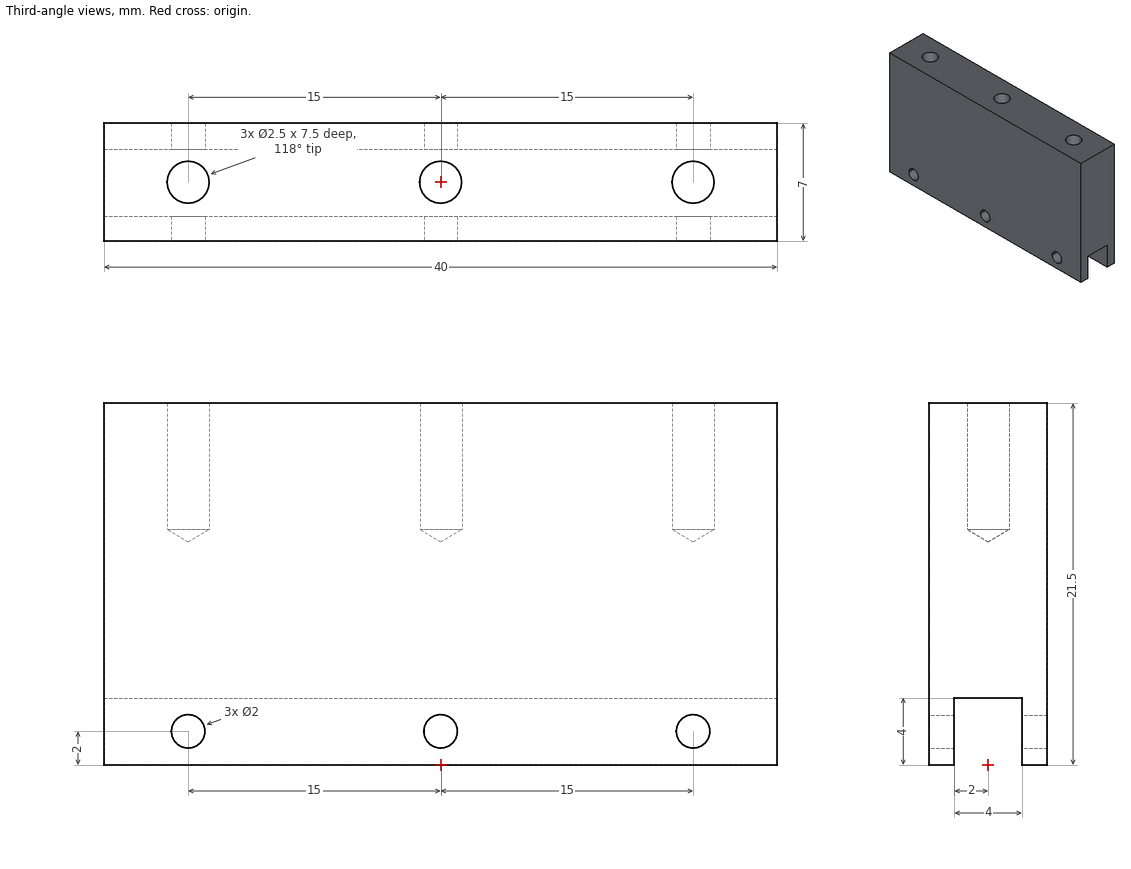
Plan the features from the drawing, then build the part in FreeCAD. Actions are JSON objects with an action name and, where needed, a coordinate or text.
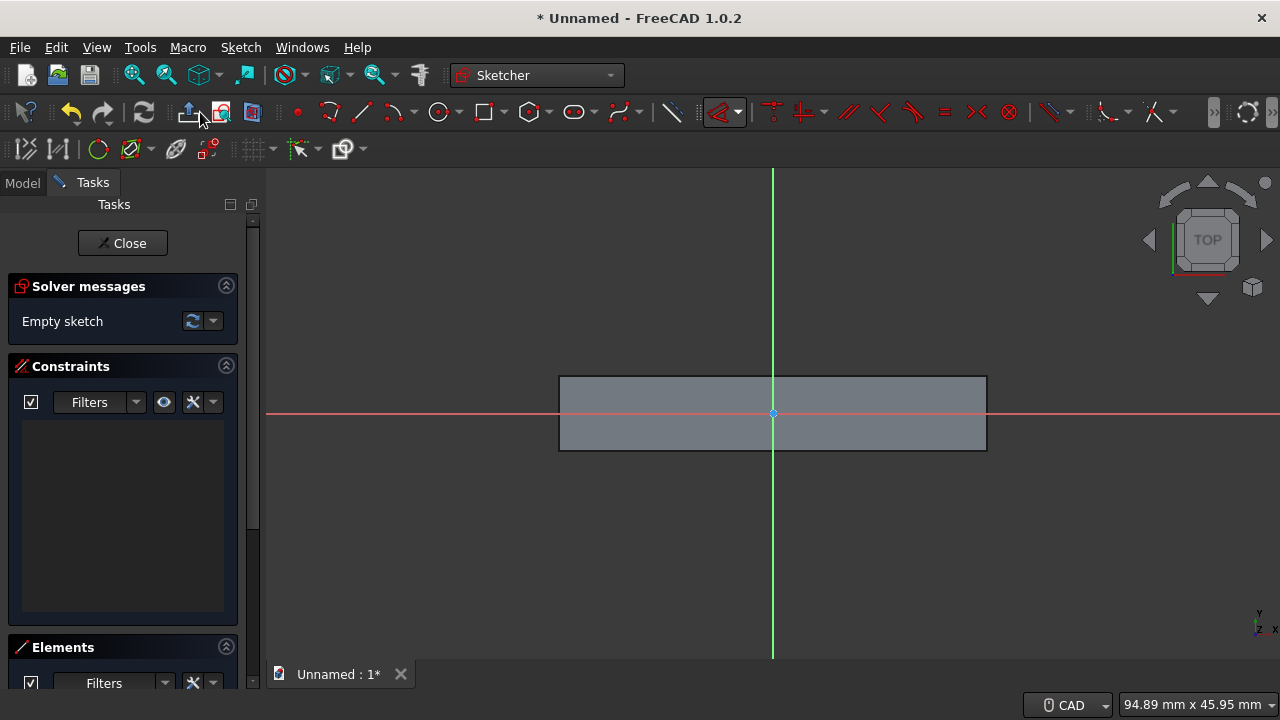
{"action": "scroll", "coordinate": [856, 414], "scroll_direction": "up", "scroll_amount": 3}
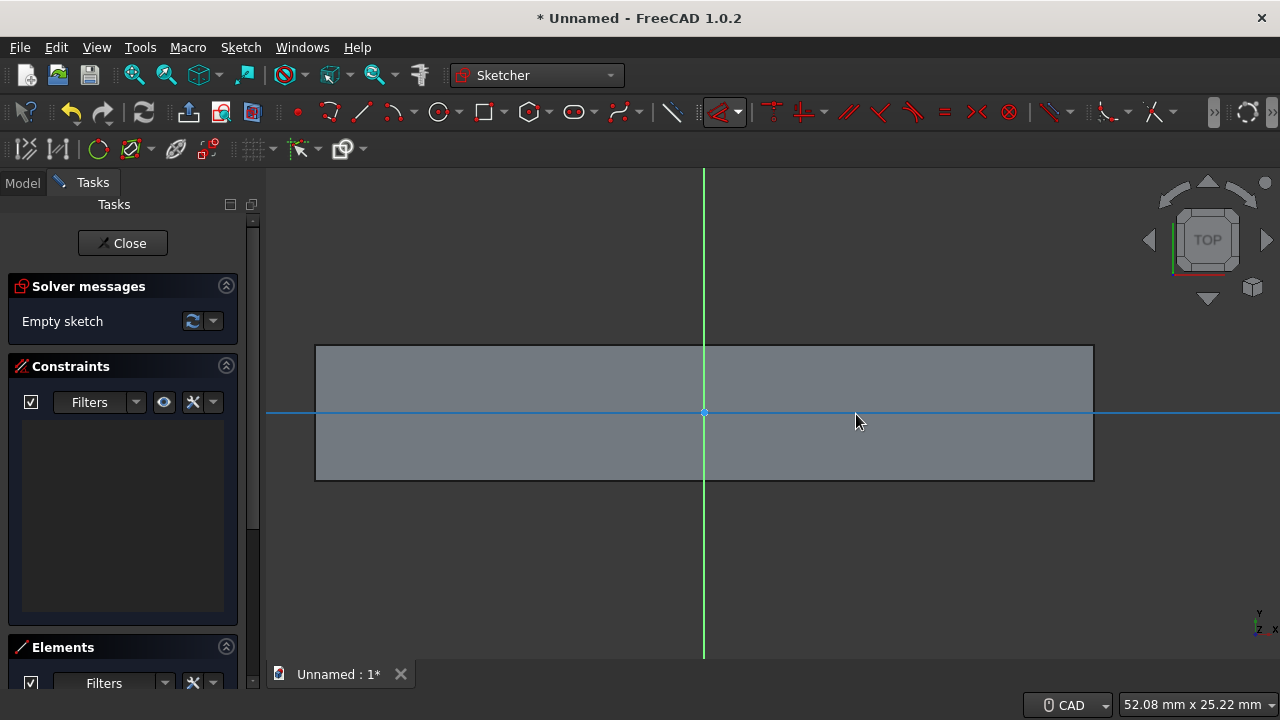
{"action": "left_click", "coordinate": [440, 112]}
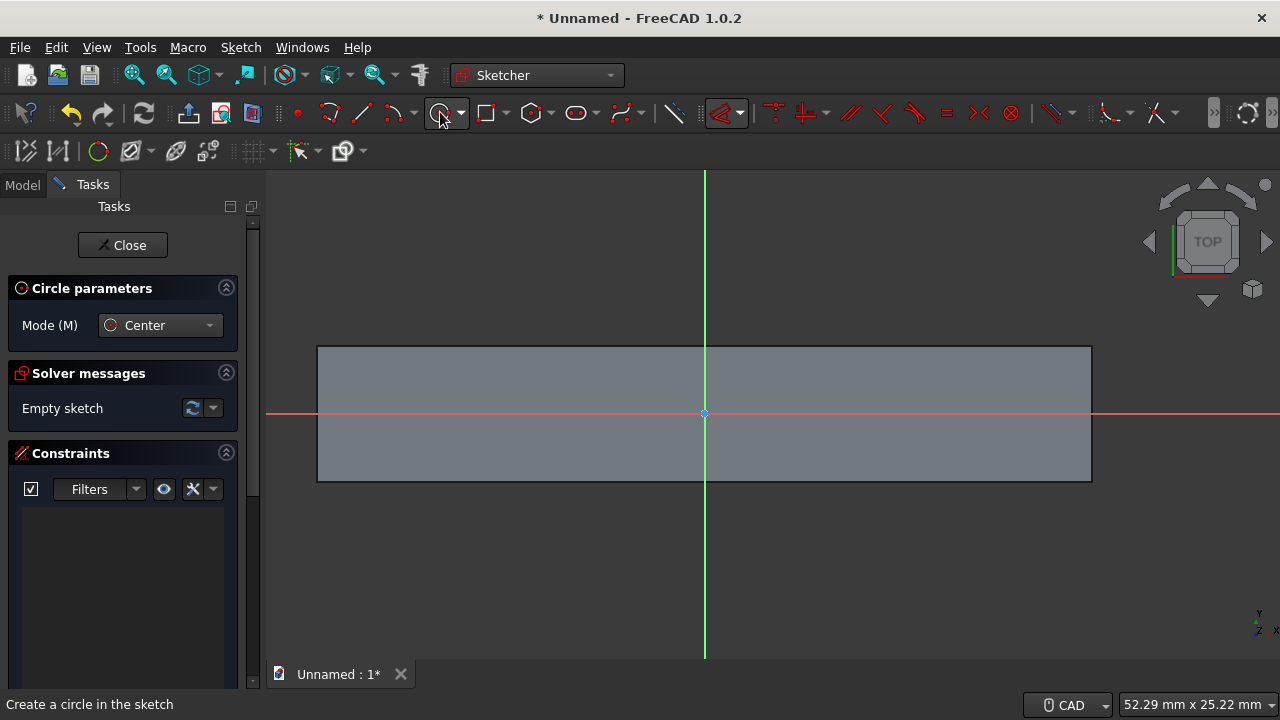
{"action": "left_click", "coordinate": [414, 414]}
{"action": "left_click", "coordinate": [431, 397]}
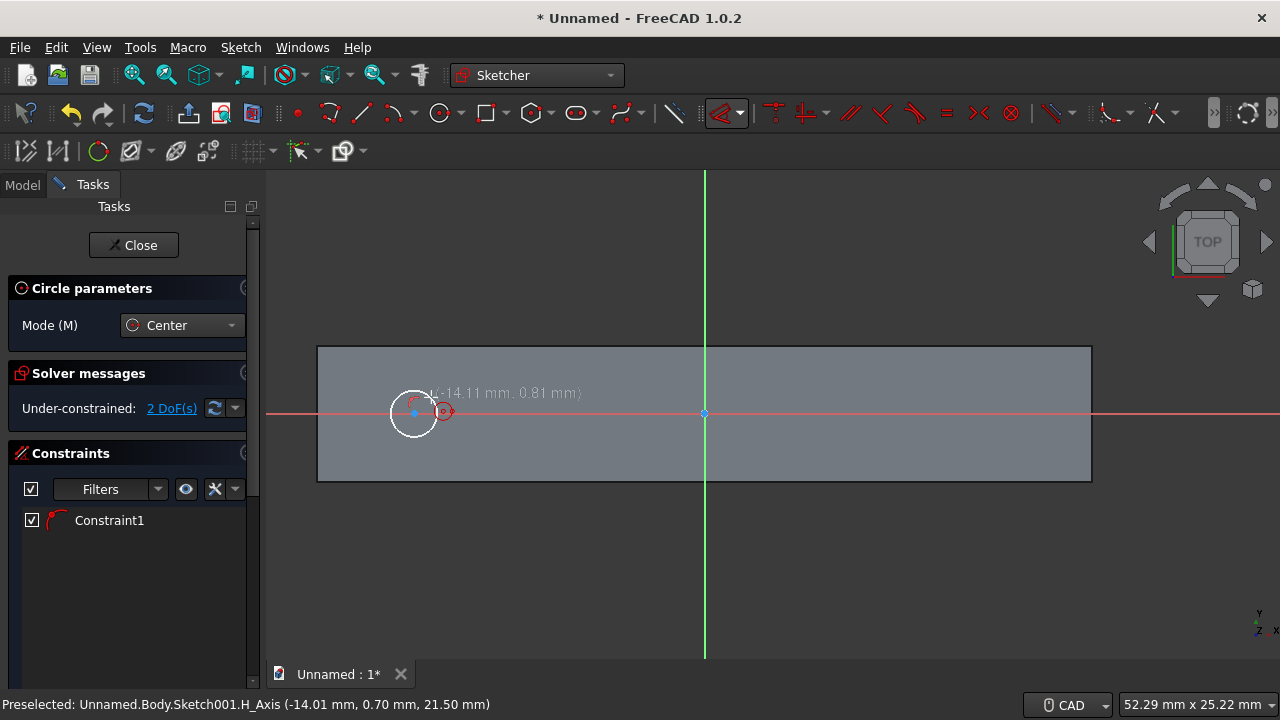
{"action": "left_click", "coordinate": [705, 414]}
{"action": "left_click", "coordinate": [722, 397]}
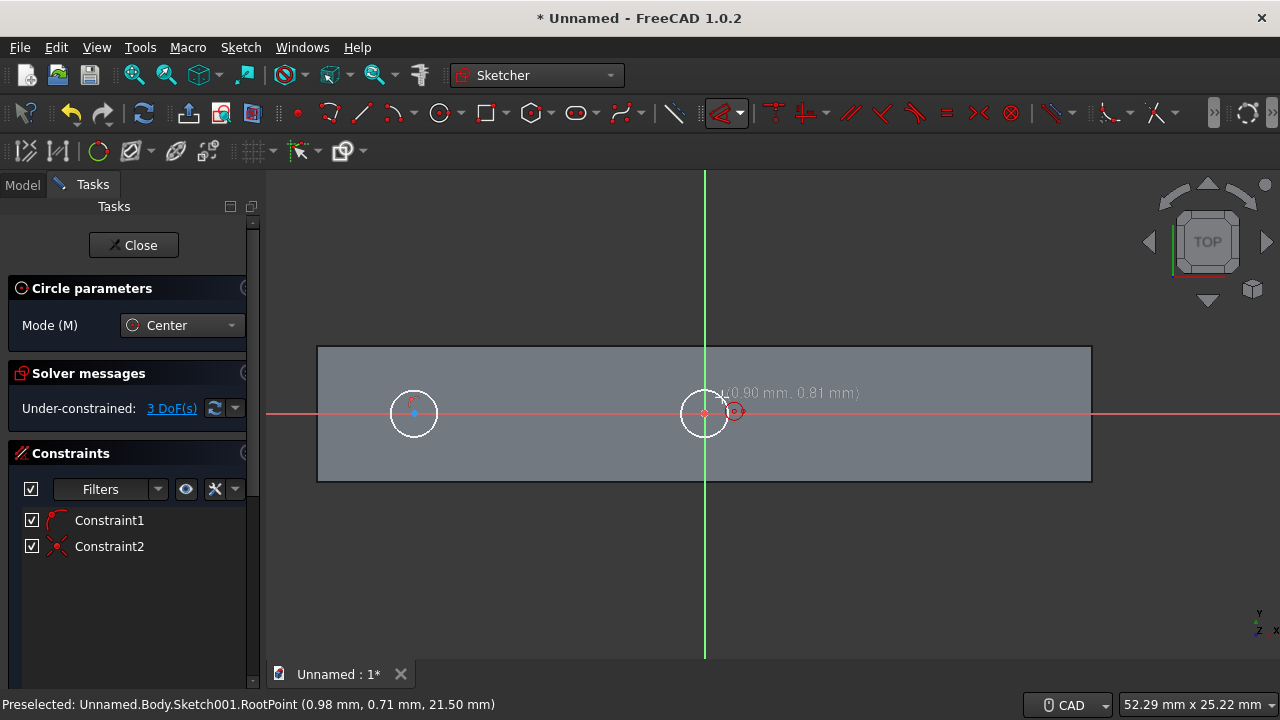
{"action": "left_click", "coordinate": [995, 414]}
{"action": "left_click", "coordinate": [1013, 397]}
{"action": "key", "text": "Escape"}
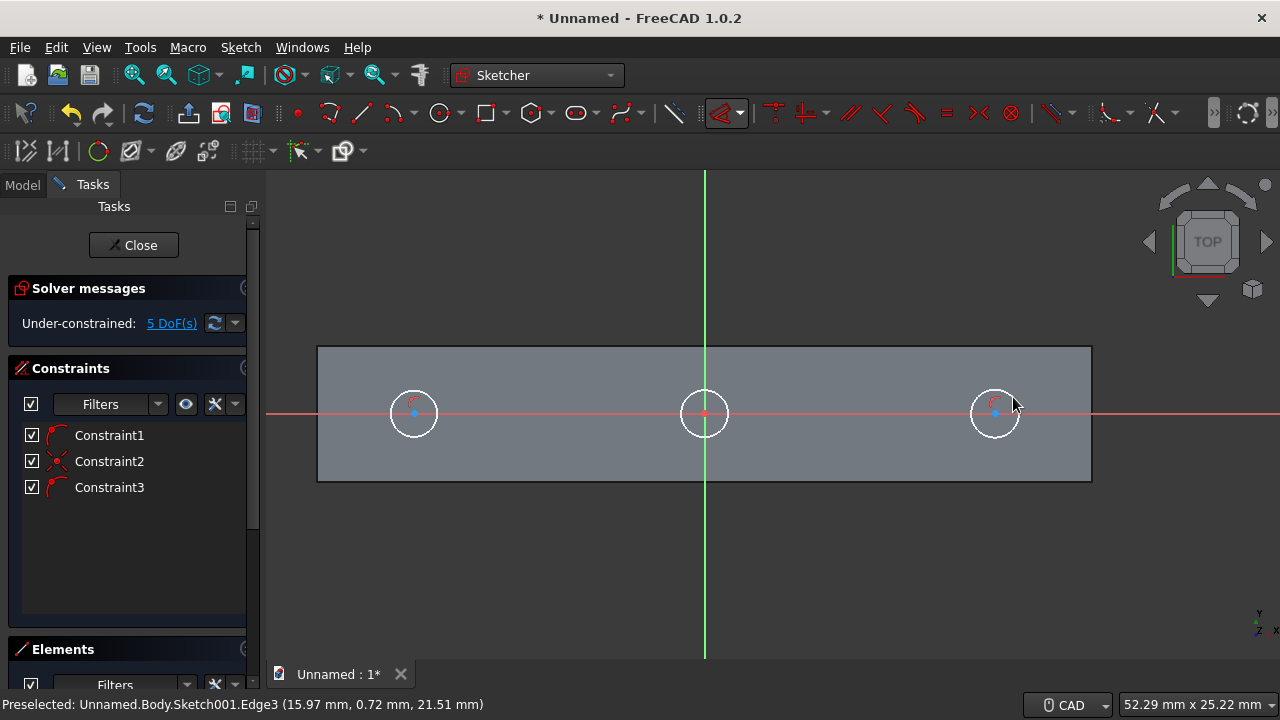
{"action": "left_click", "coordinate": [430, 397]}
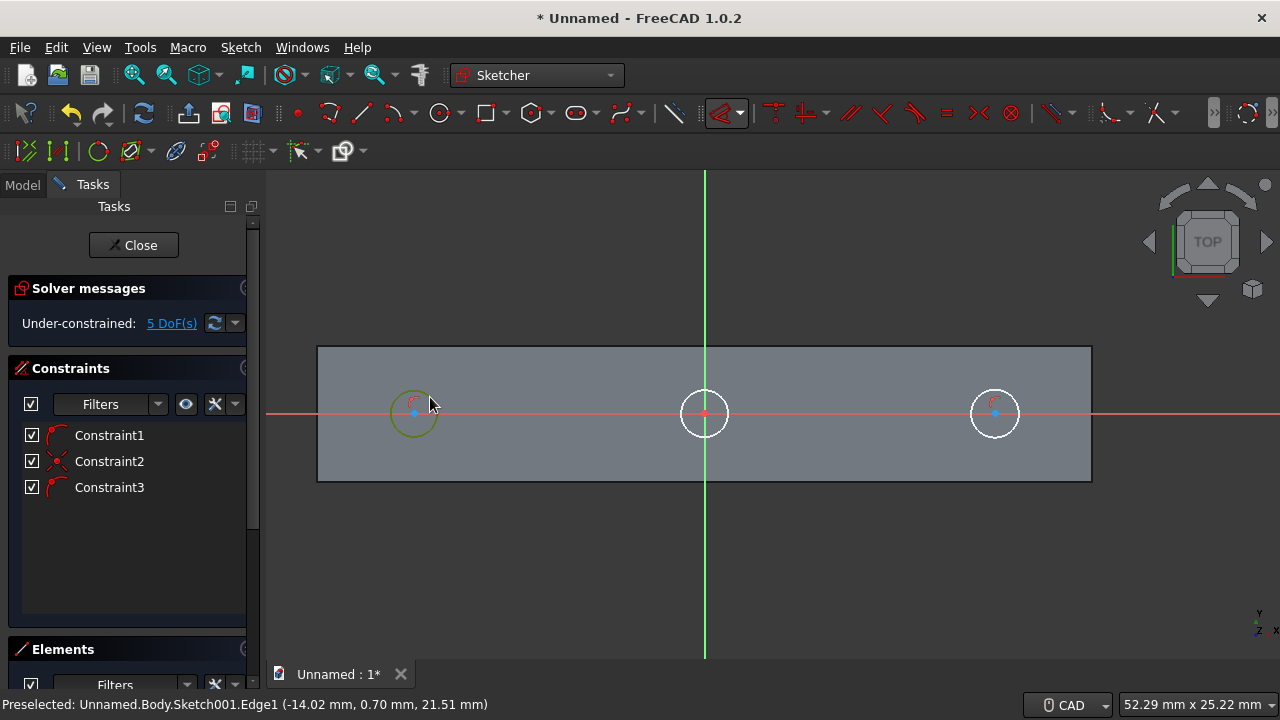
{"action": "left_click", "coordinate": [721, 397]}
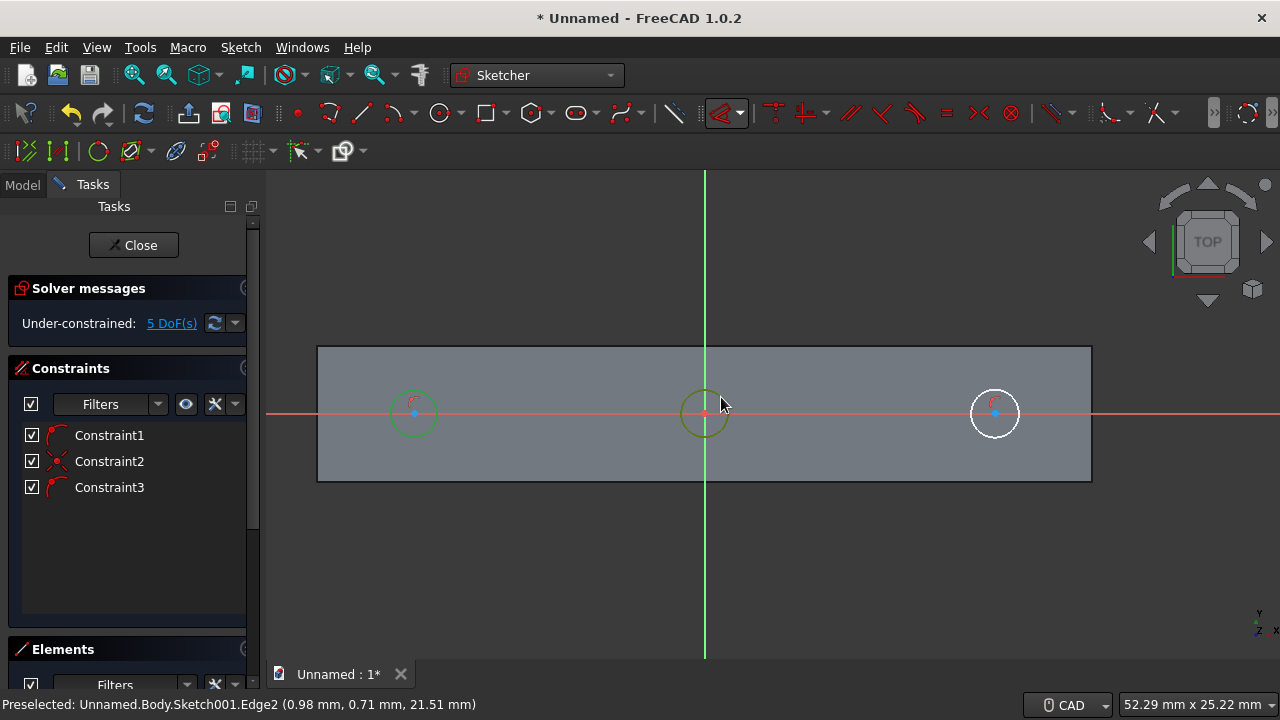
{"action": "left_click", "coordinate": [1012, 397]}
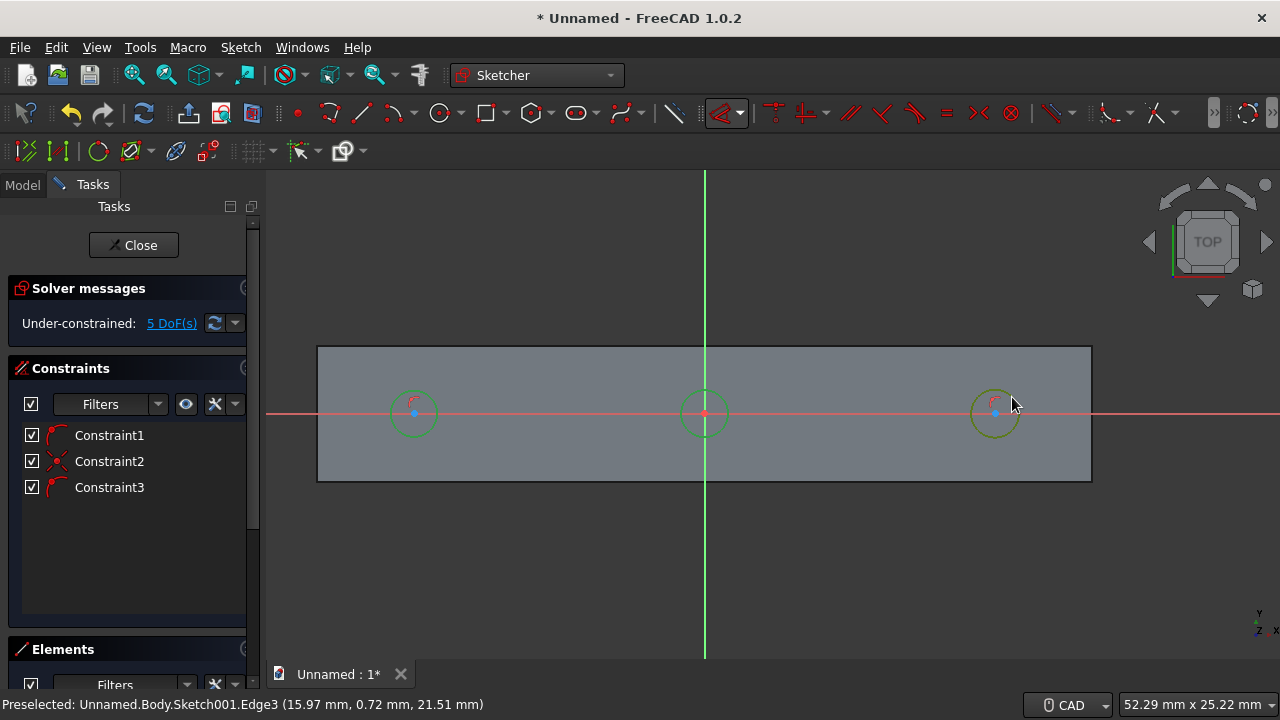
{"action": "left_click", "coordinate": [948, 114]}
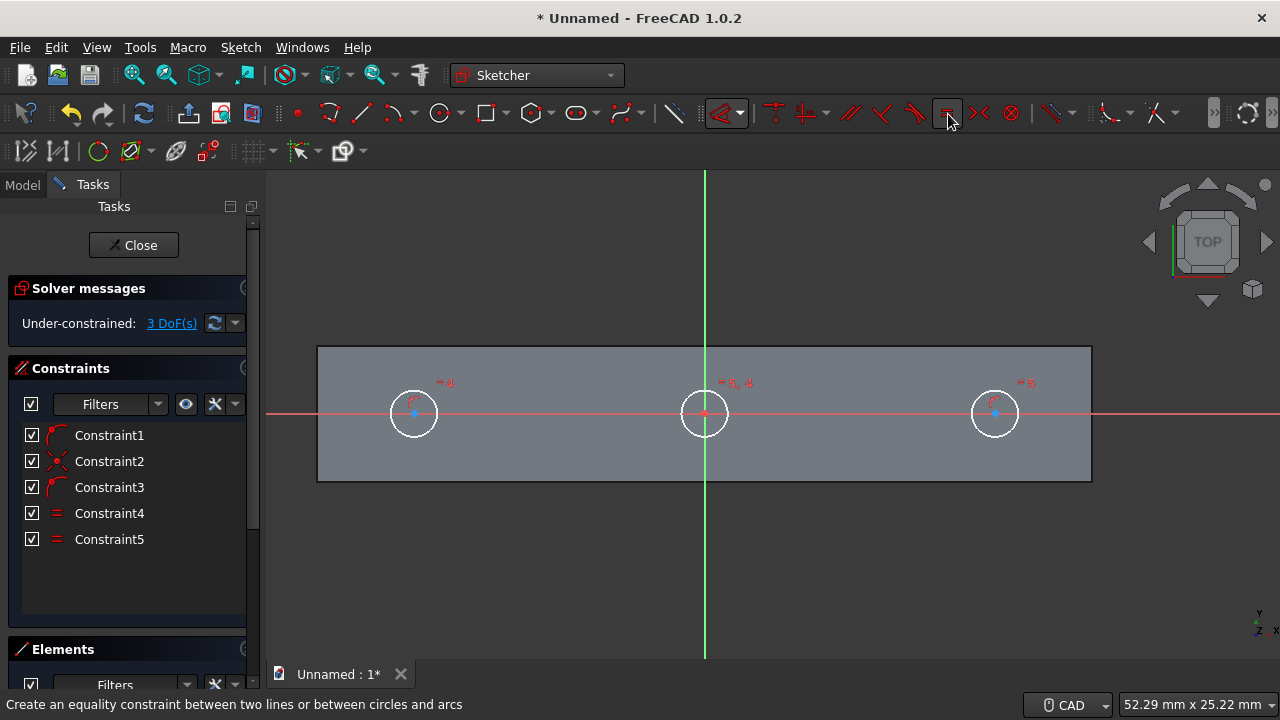
{"action": "left_click", "coordinate": [430, 397]}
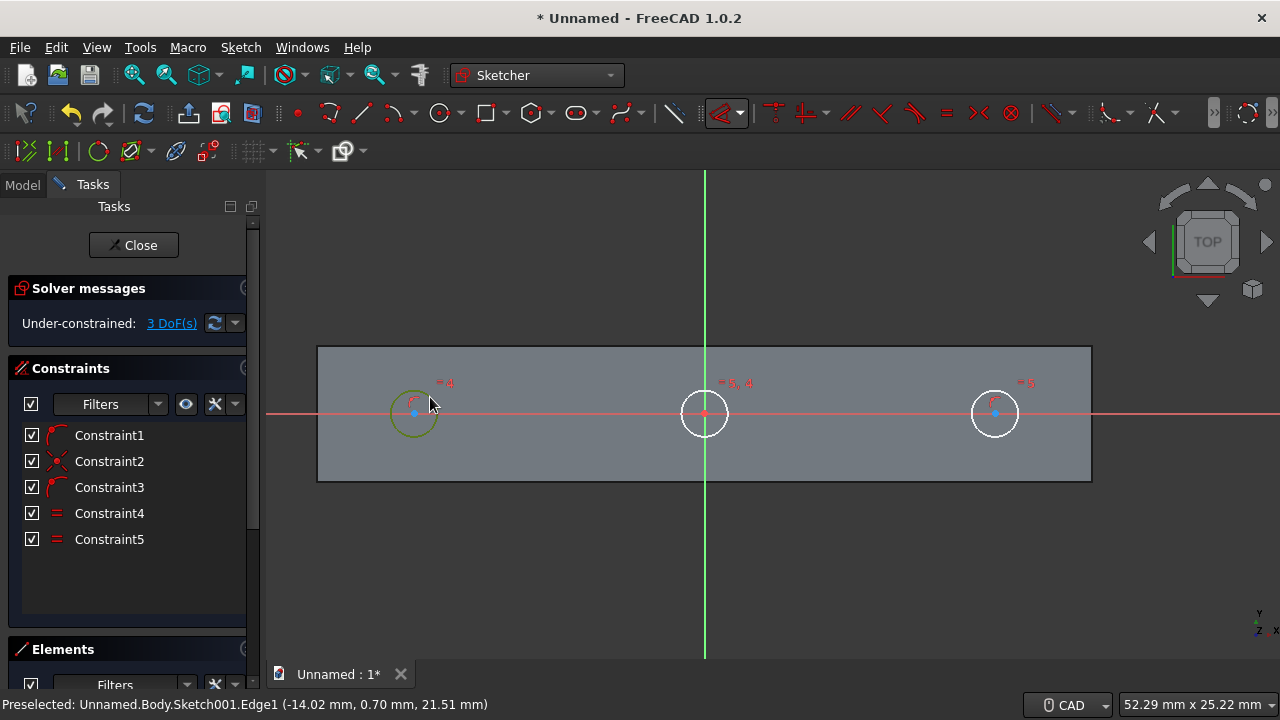
{"action": "left_click", "coordinate": [742, 114]}